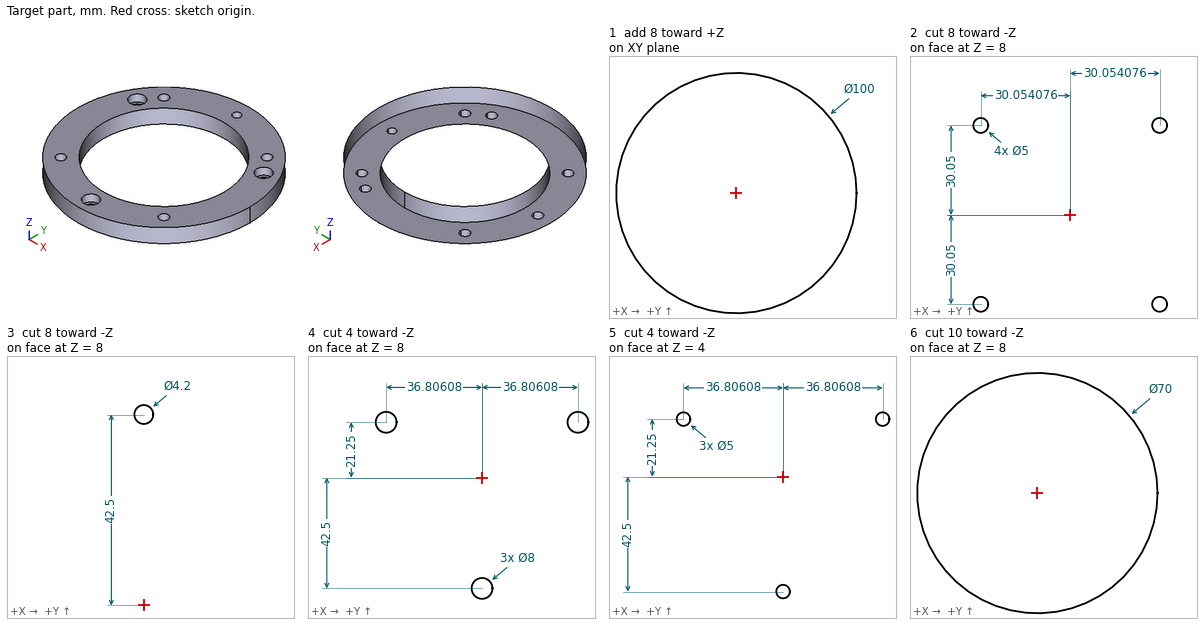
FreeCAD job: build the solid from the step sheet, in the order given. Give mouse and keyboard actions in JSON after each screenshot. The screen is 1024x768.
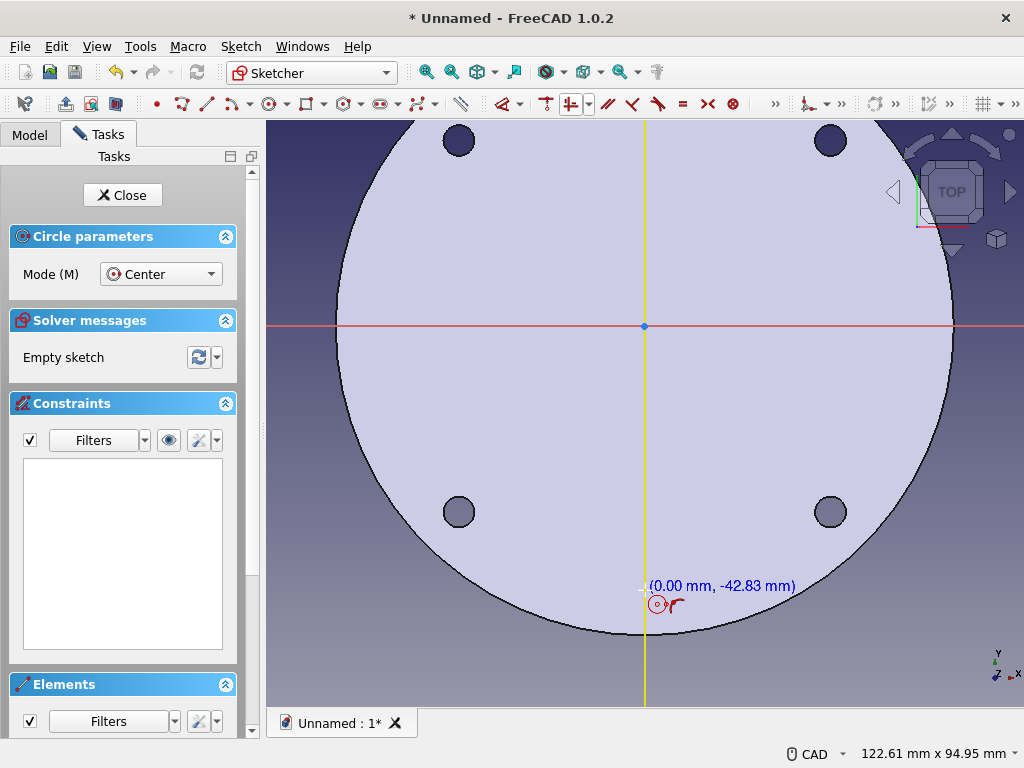
{"action": "left_click", "coordinate": [645, 589]}
{"action": "mouse_move", "coordinate": [662, 572]}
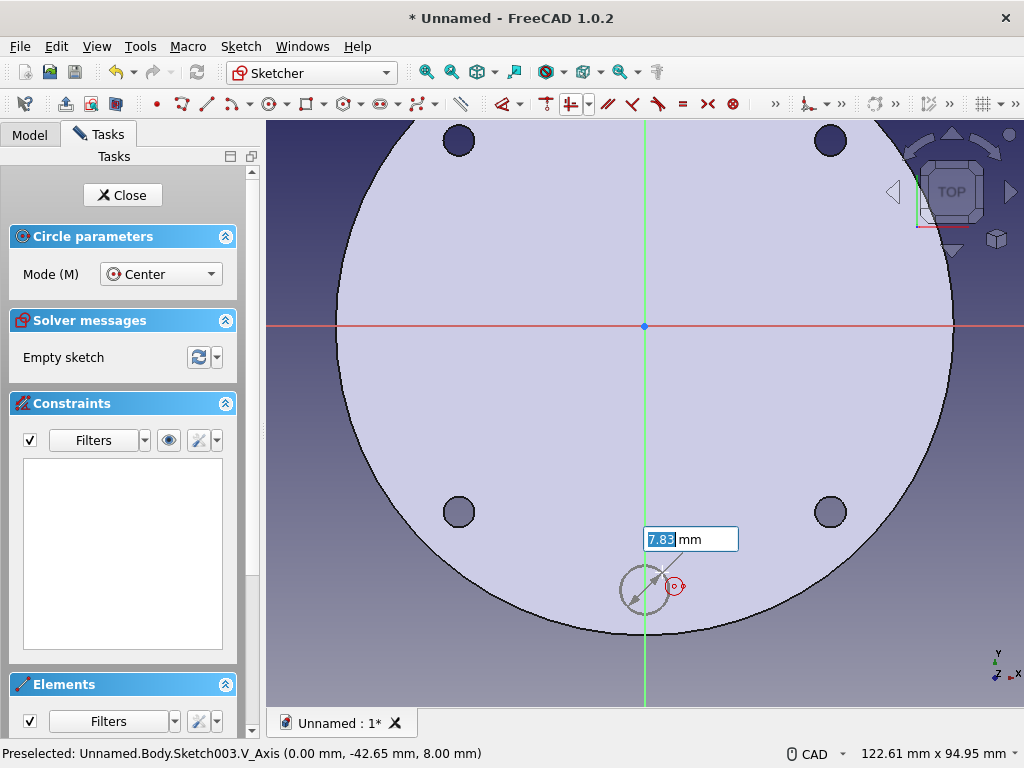
{"action": "type", "text": "8"}
{"action": "key", "text": "Return"}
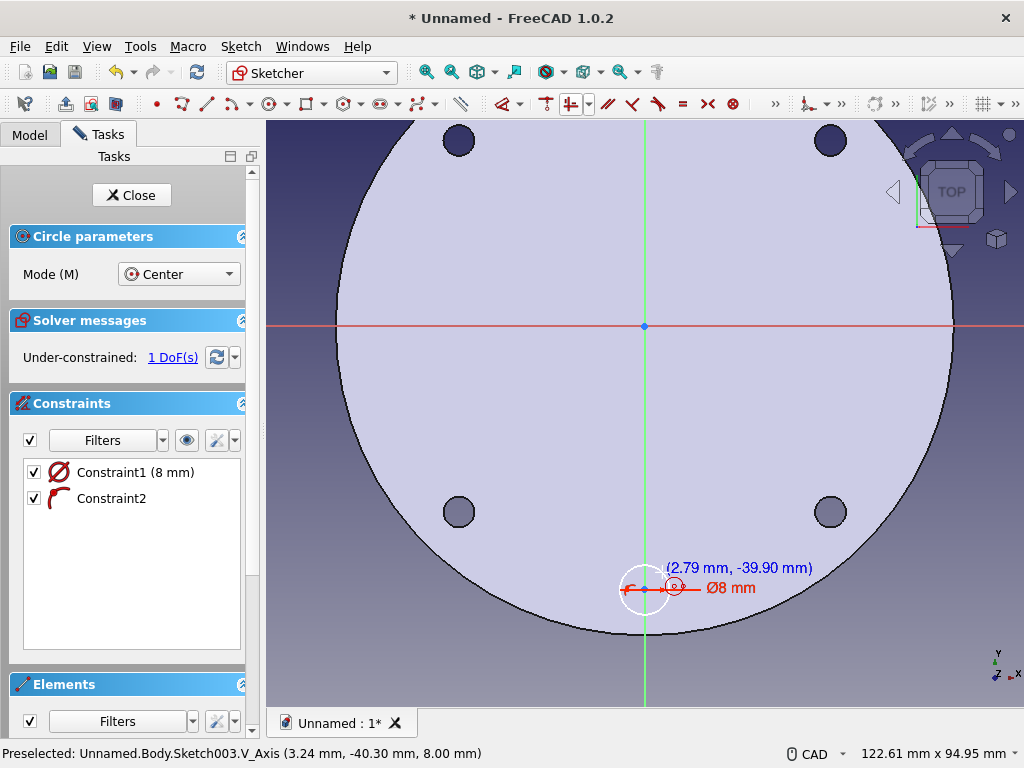
{"action": "left_click", "coordinate": [417, 195]}
{"action": "mouse_move", "coordinate": [435, 177]}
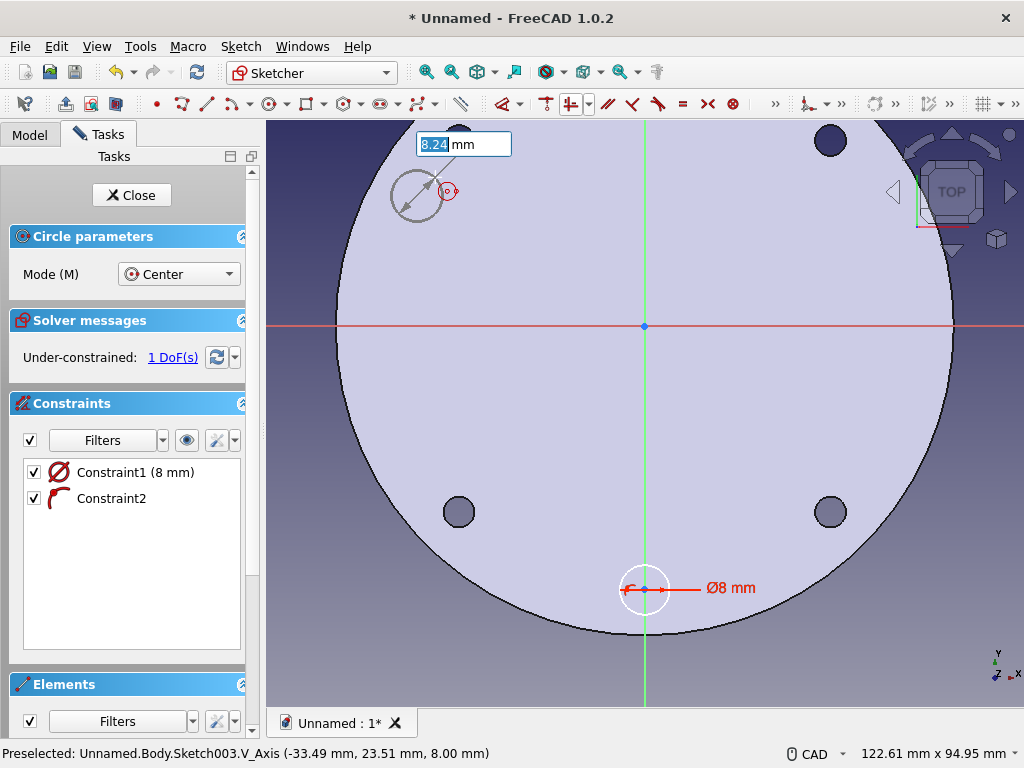
{"action": "type", "text": "8"}
{"action": "key", "text": "Return"}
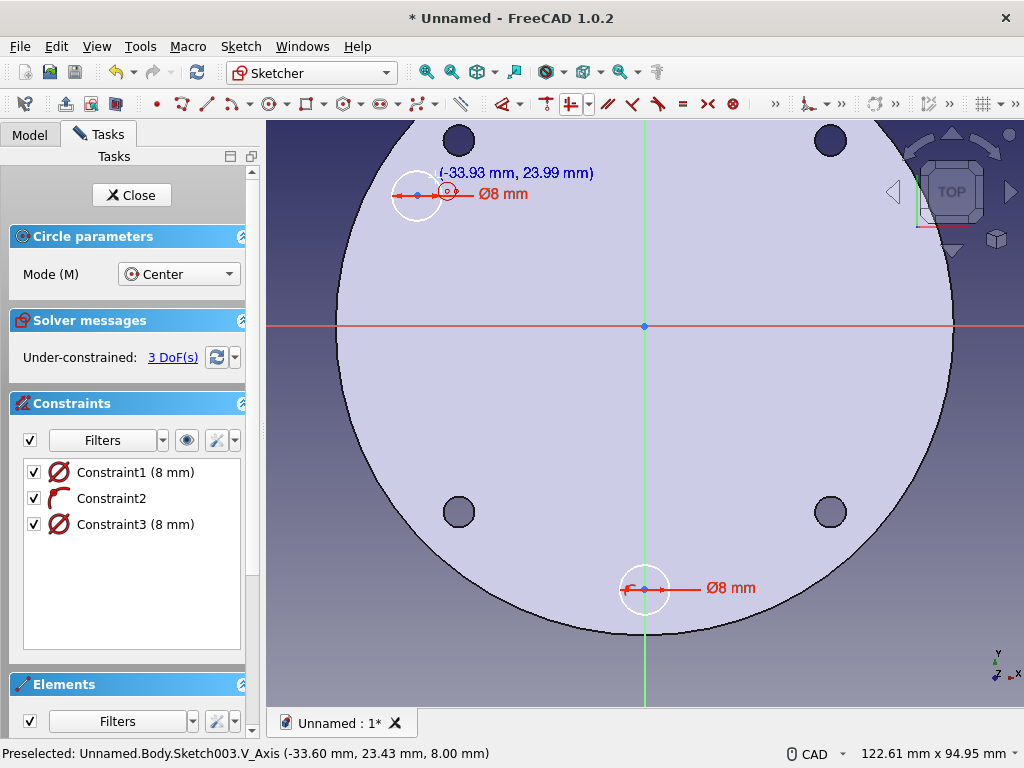
{"action": "scroll", "coordinate": [294, 511], "scroll_direction": "down", "scroll_amount": 1}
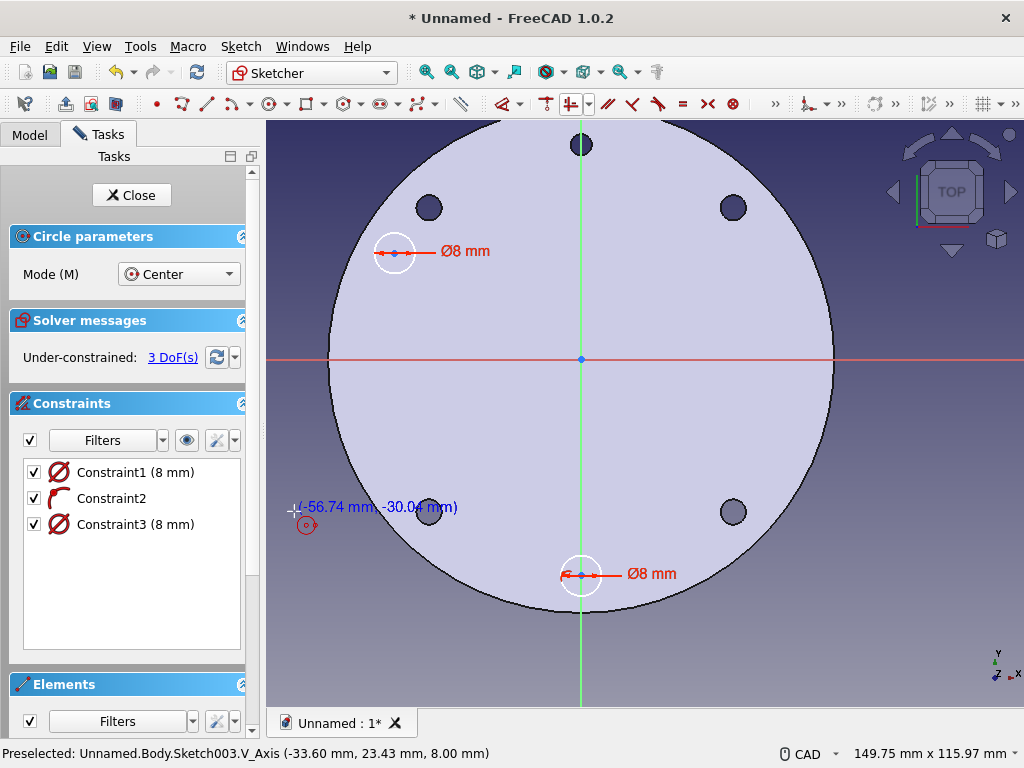
{"action": "left_click", "coordinate": [767, 252]}
{"action": "mouse_move", "coordinate": [782, 238]}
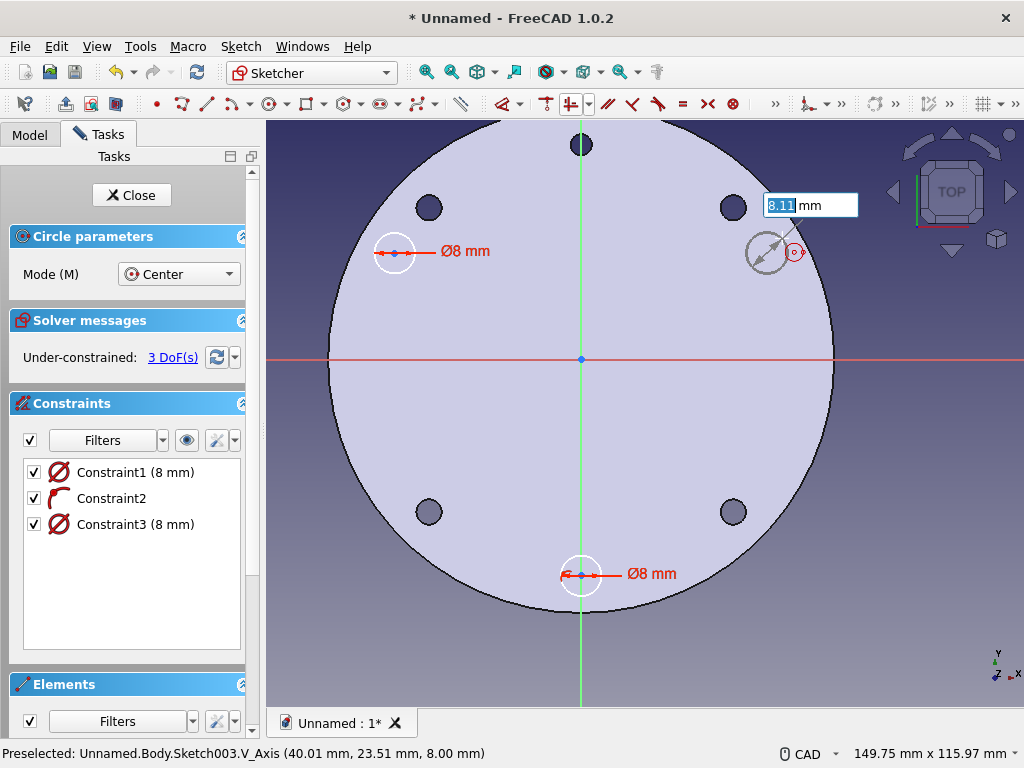
{"action": "type", "text": "8"}
{"action": "key", "text": "Return"}
{"action": "key", "text": "Escape"}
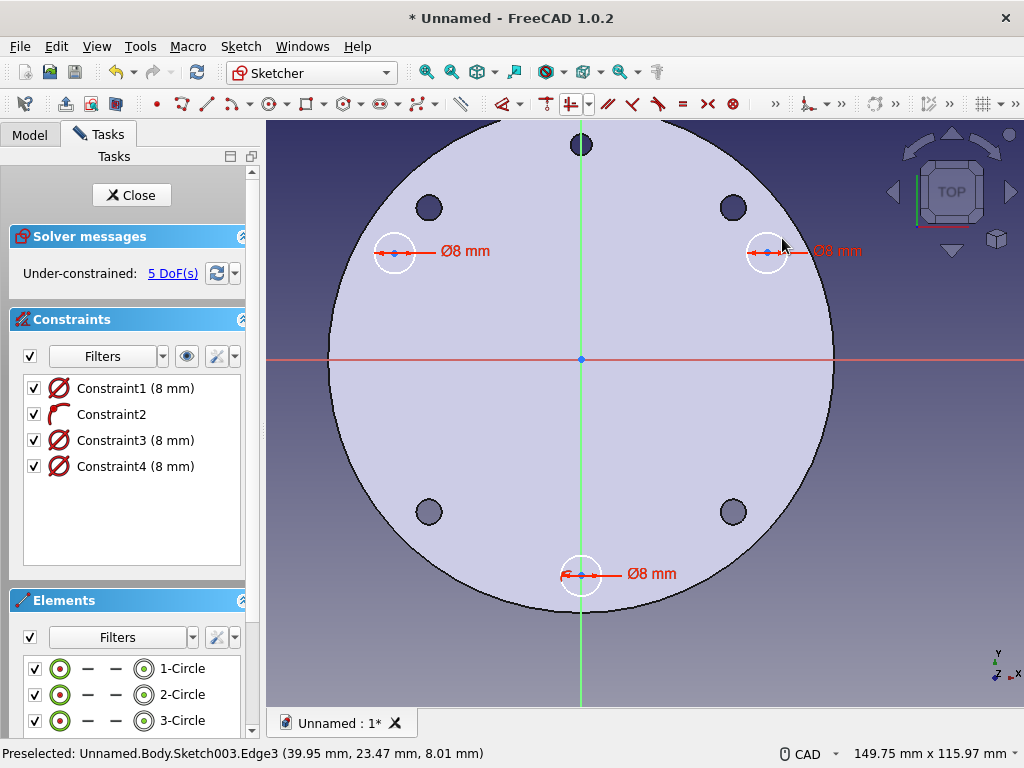
{"action": "left_click", "coordinate": [395, 253]}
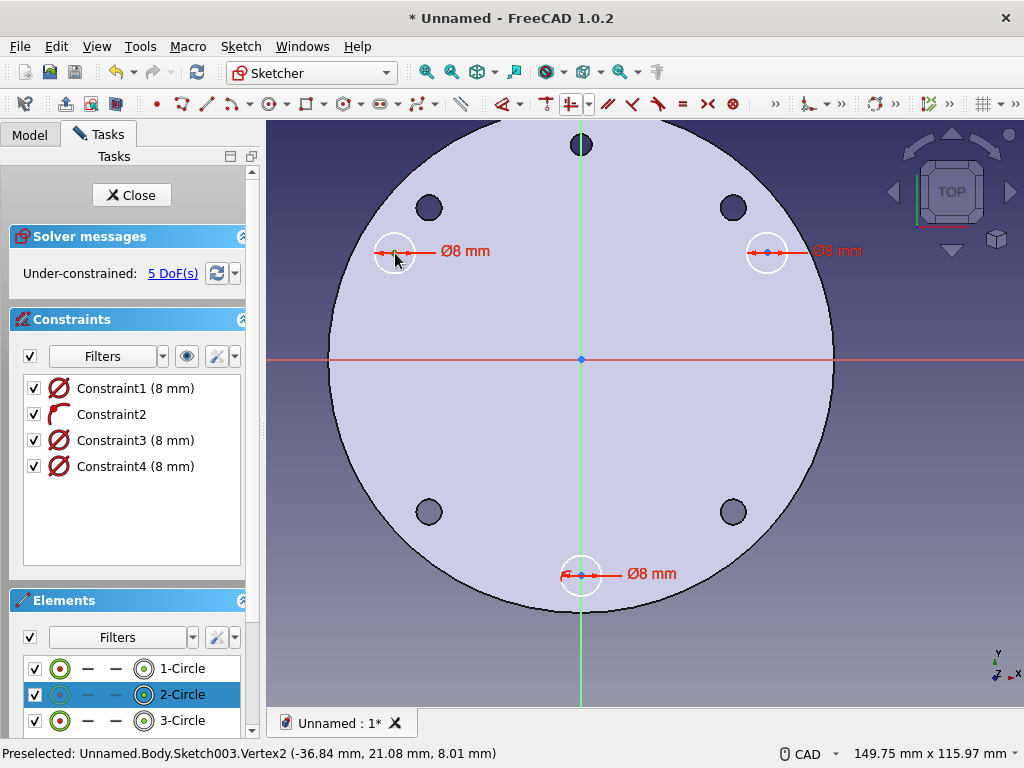
{"action": "left_click", "coordinate": [767, 253]}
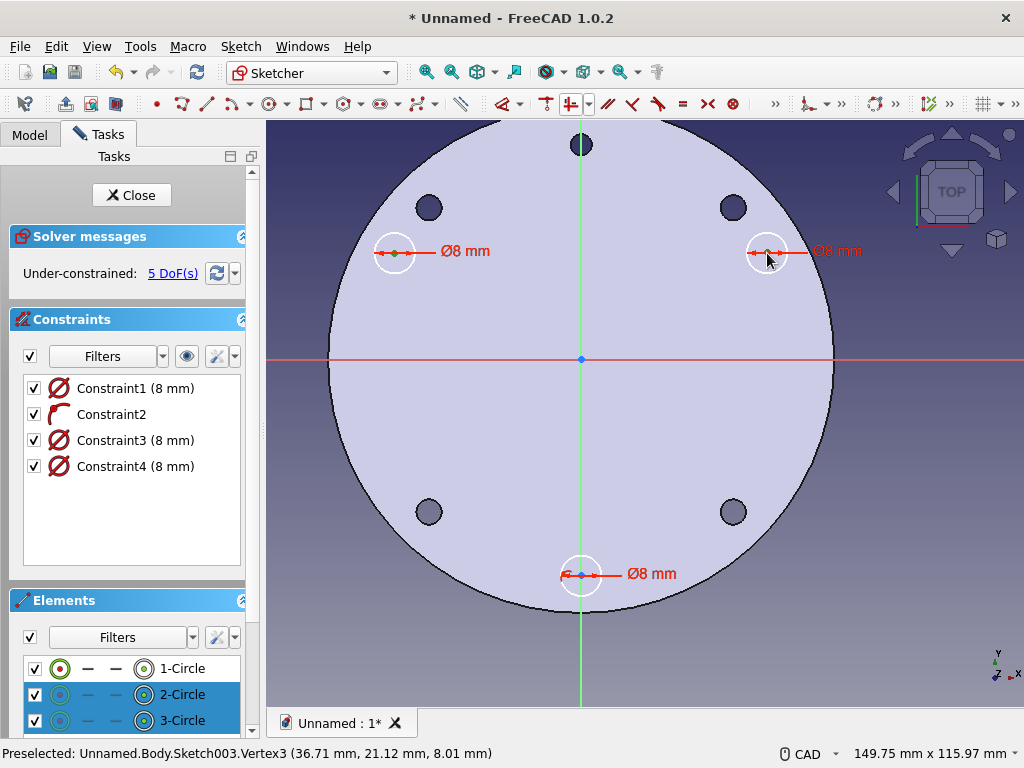
{"action": "left_click", "coordinate": [588, 104]}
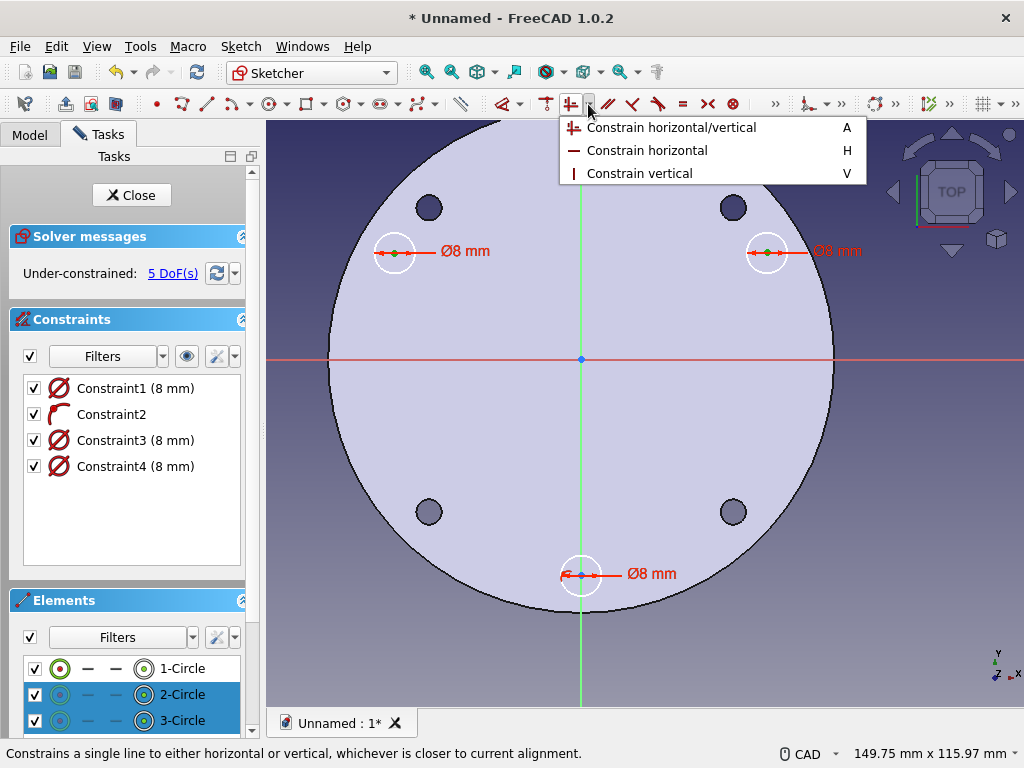
{"action": "left_click", "coordinate": [713, 150]}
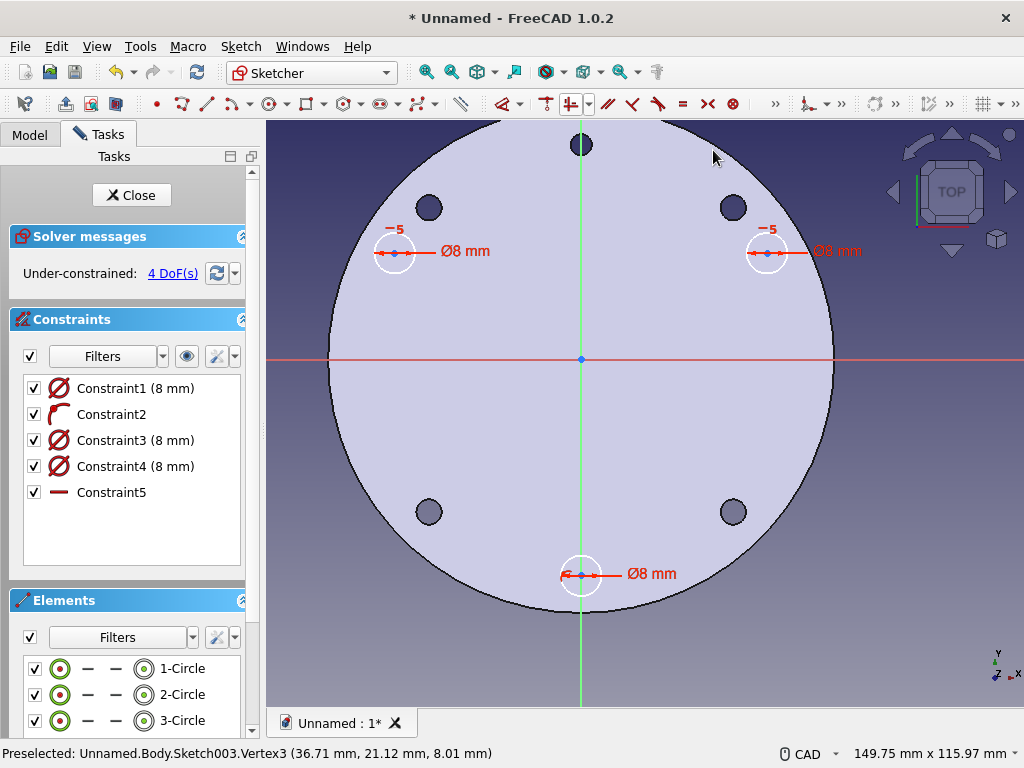
{"action": "key", "text": "d"}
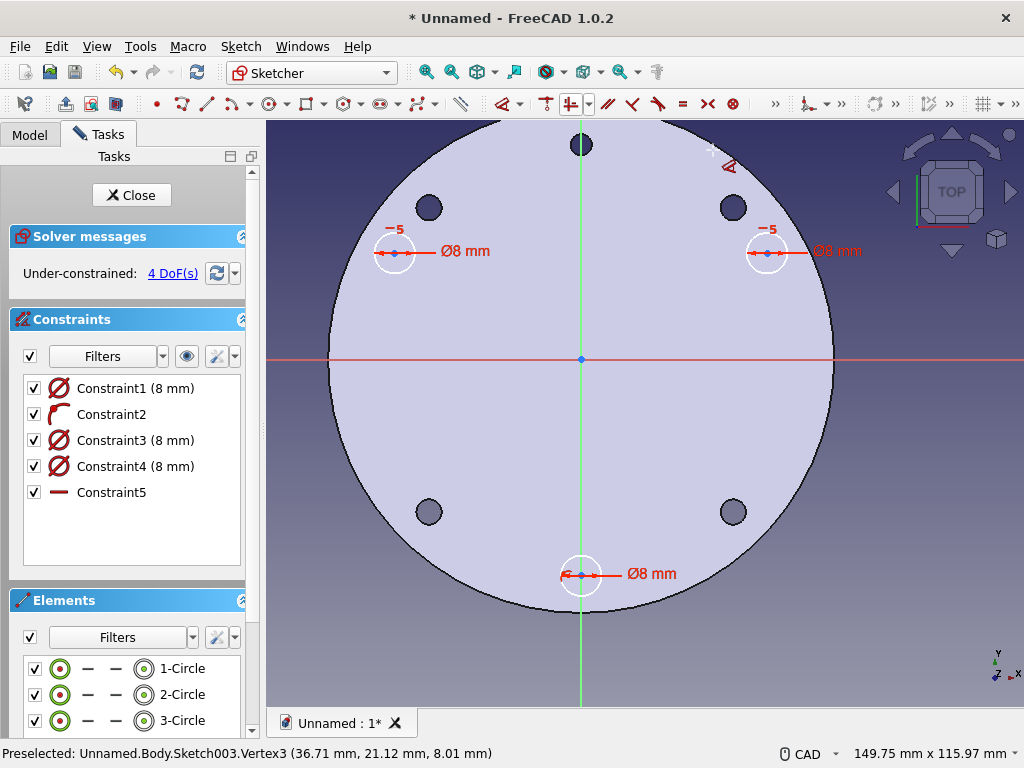
{"action": "left_click", "coordinate": [581, 576]}
{"action": "left_click", "coordinate": [615, 468]}